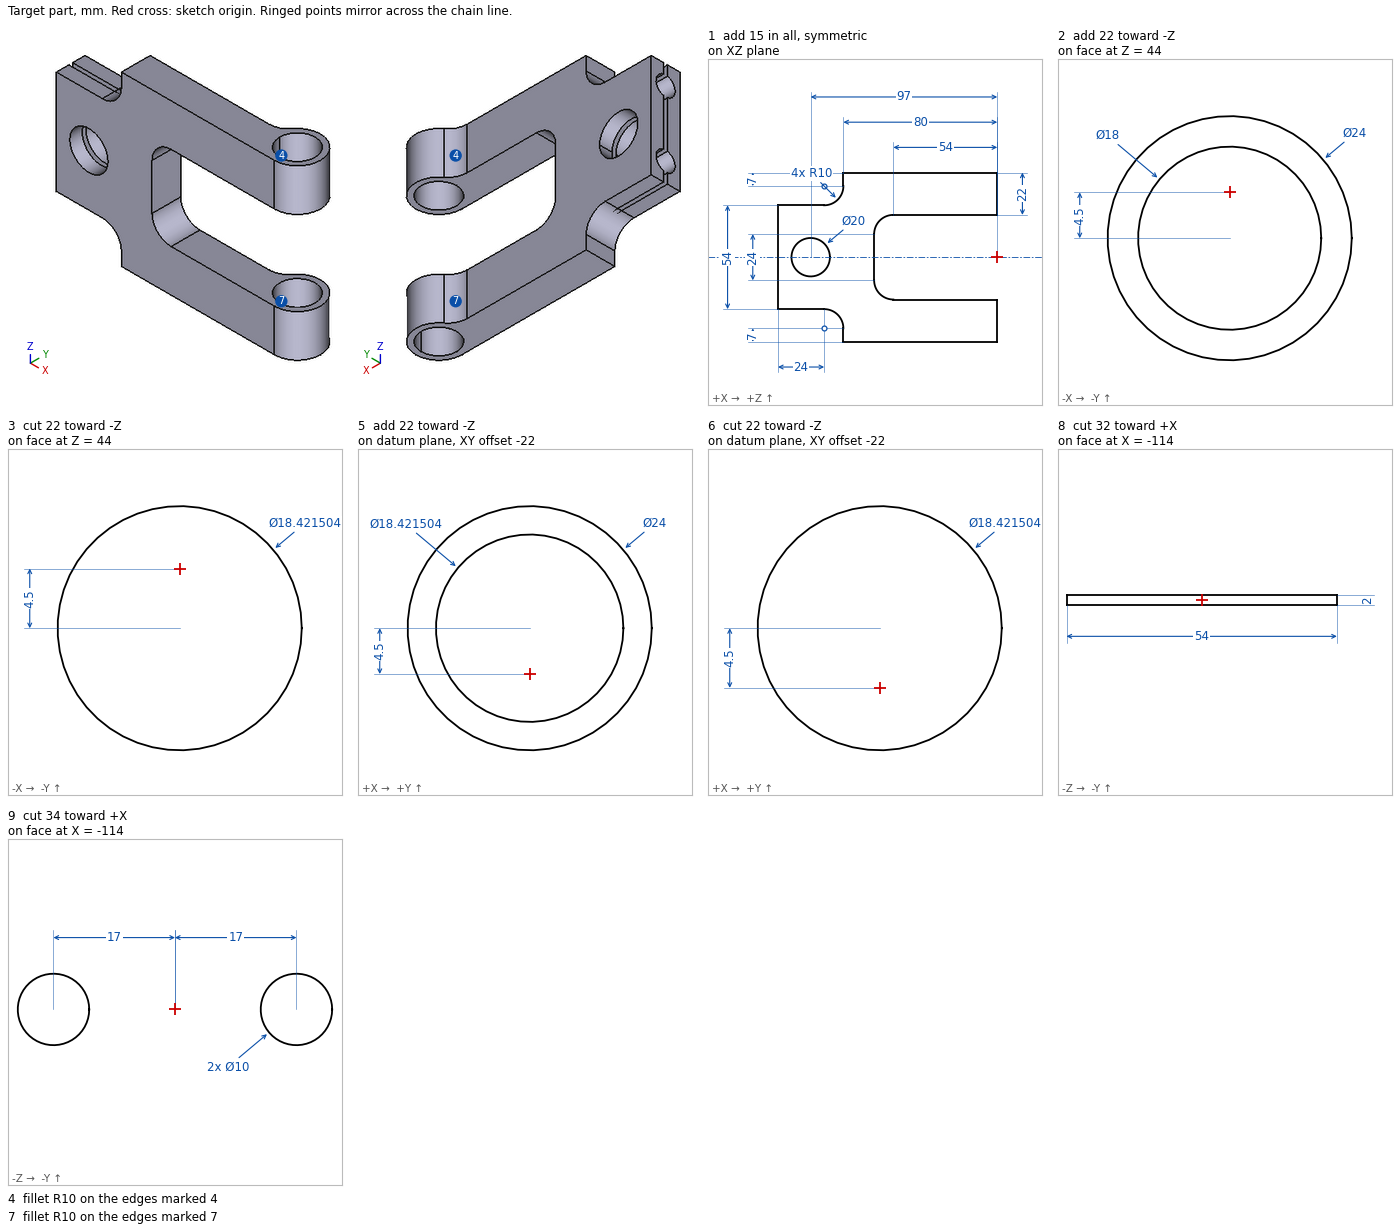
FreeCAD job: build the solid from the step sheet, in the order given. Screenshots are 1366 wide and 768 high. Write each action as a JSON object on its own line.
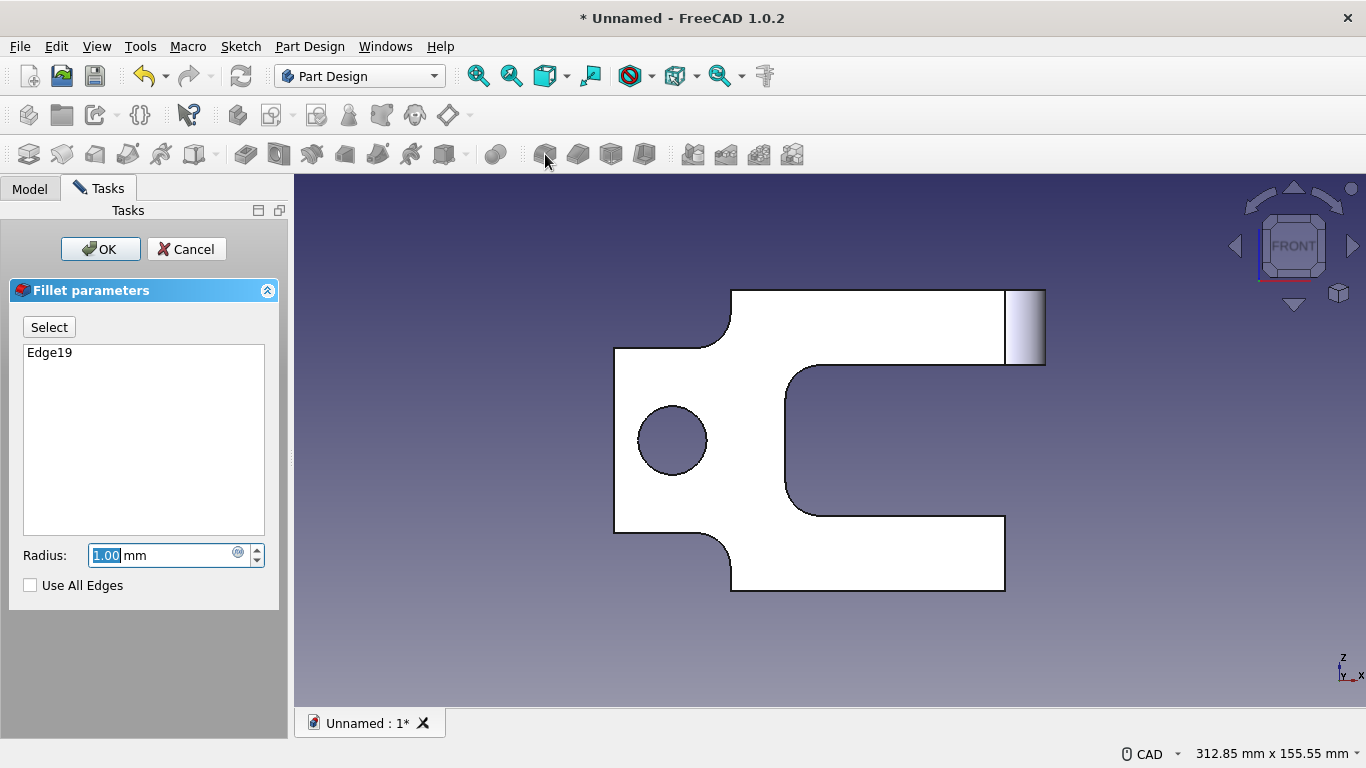
{"action": "type", "text": "10"}
{"action": "key", "text": "Tab"}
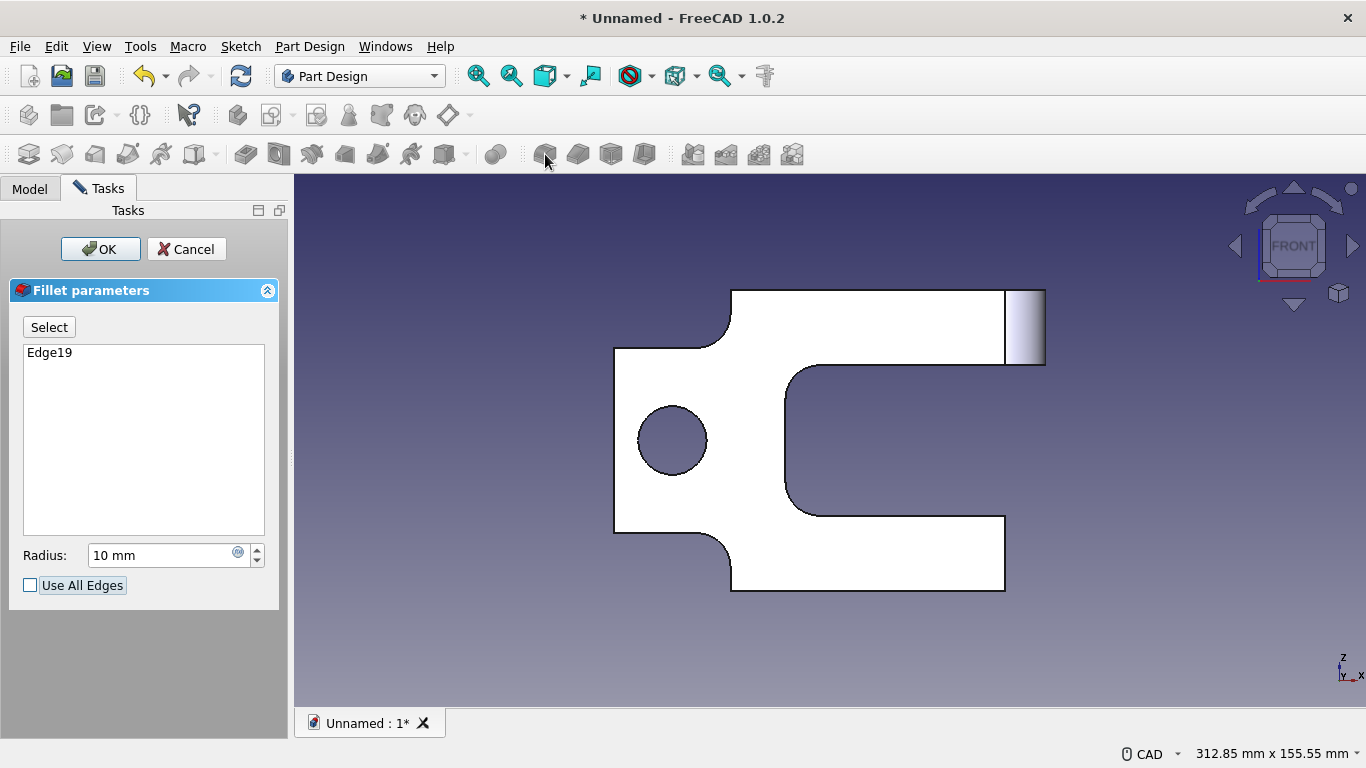
{"action": "left_click", "coordinate": [101, 249]}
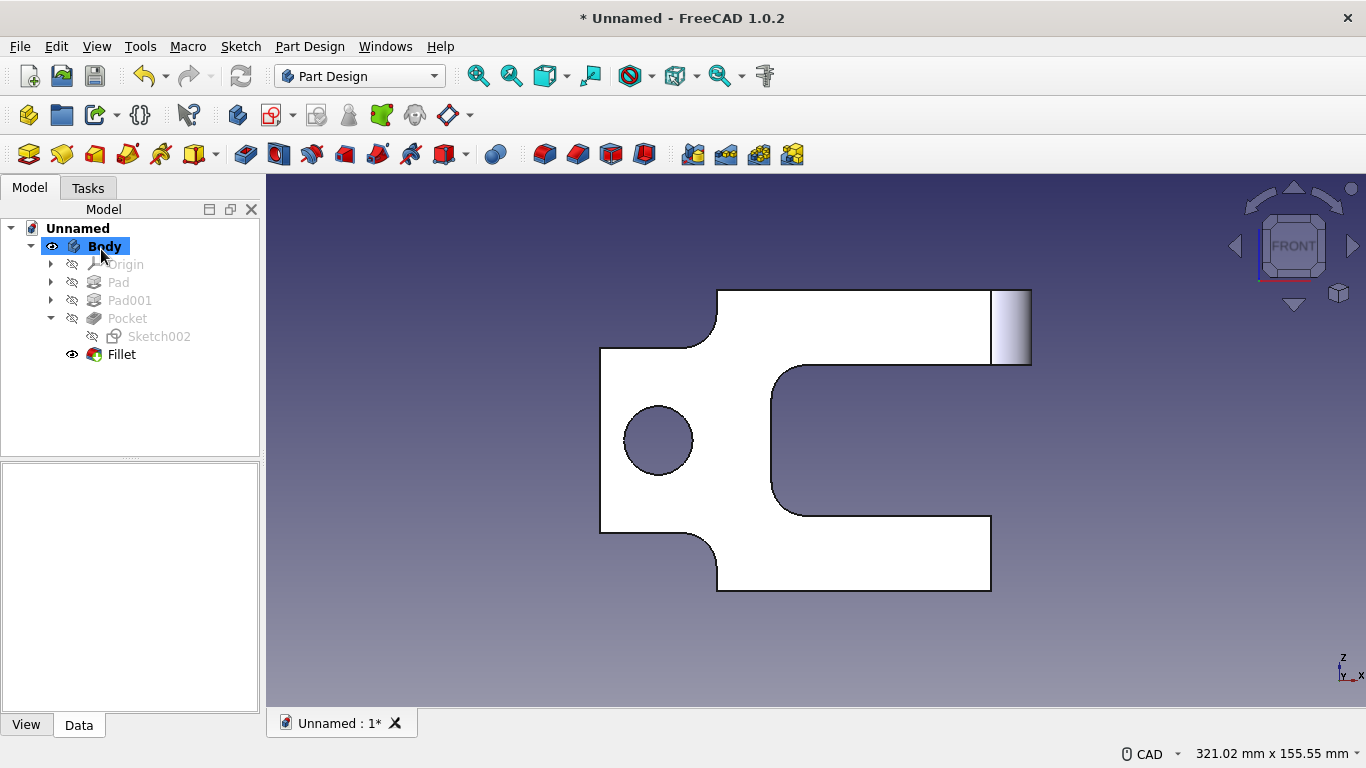
{"action": "left_click", "coordinate": [51, 264]}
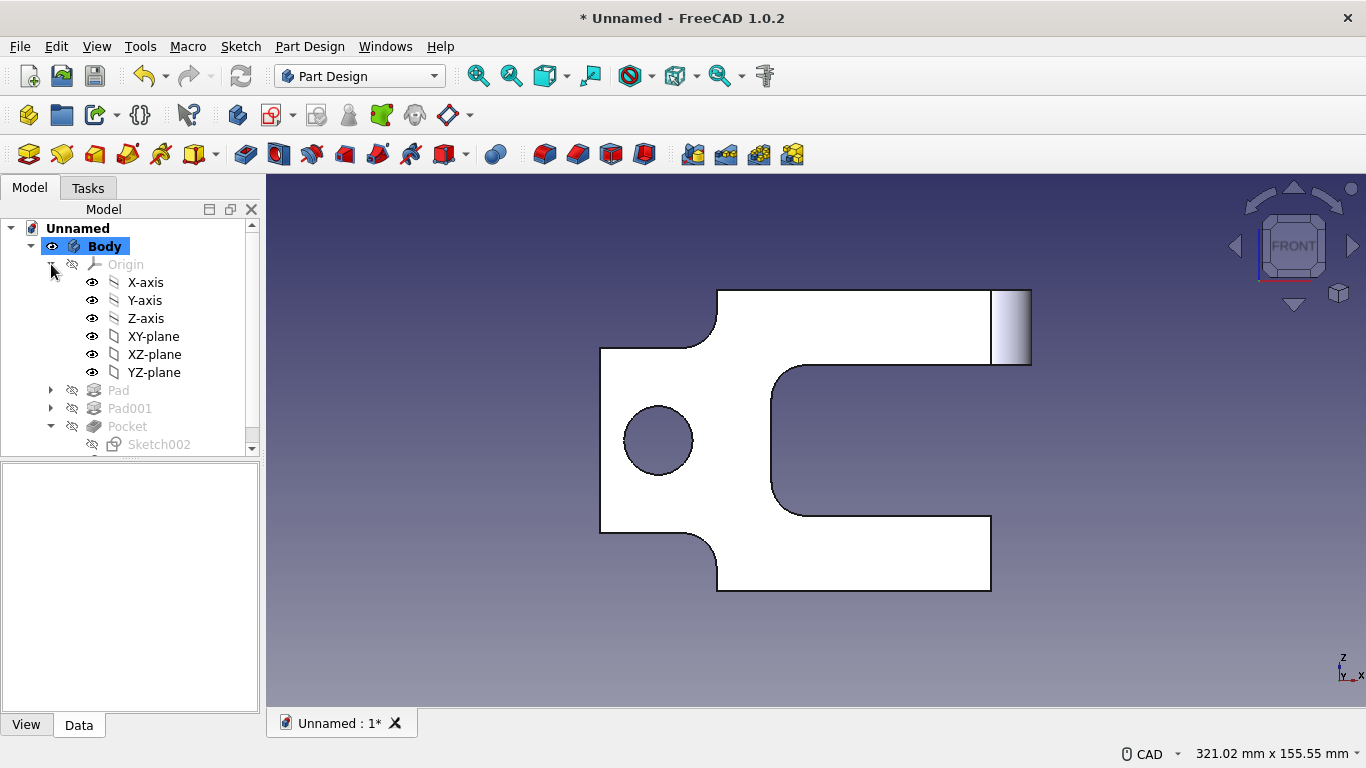
{"action": "left_click", "coordinate": [137, 336]}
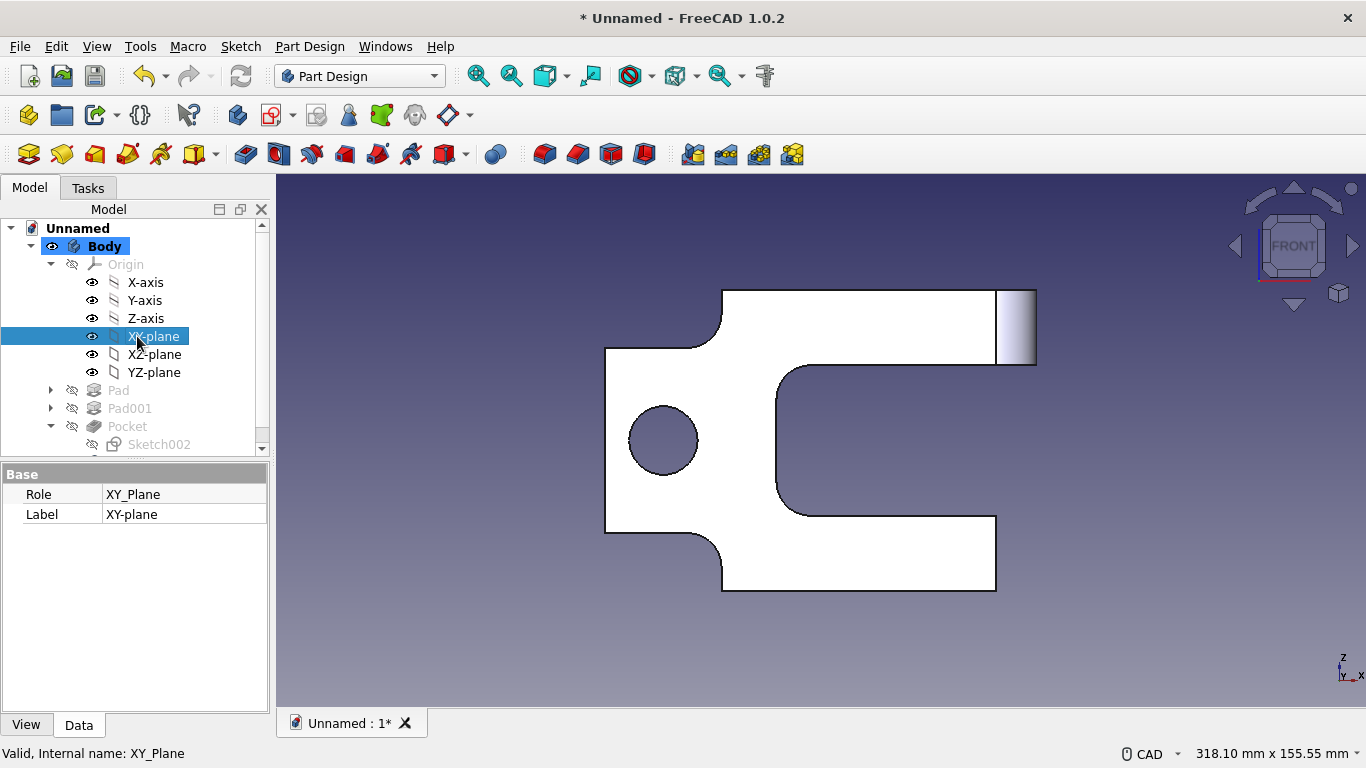
{"action": "left_click", "coordinate": [448, 116]}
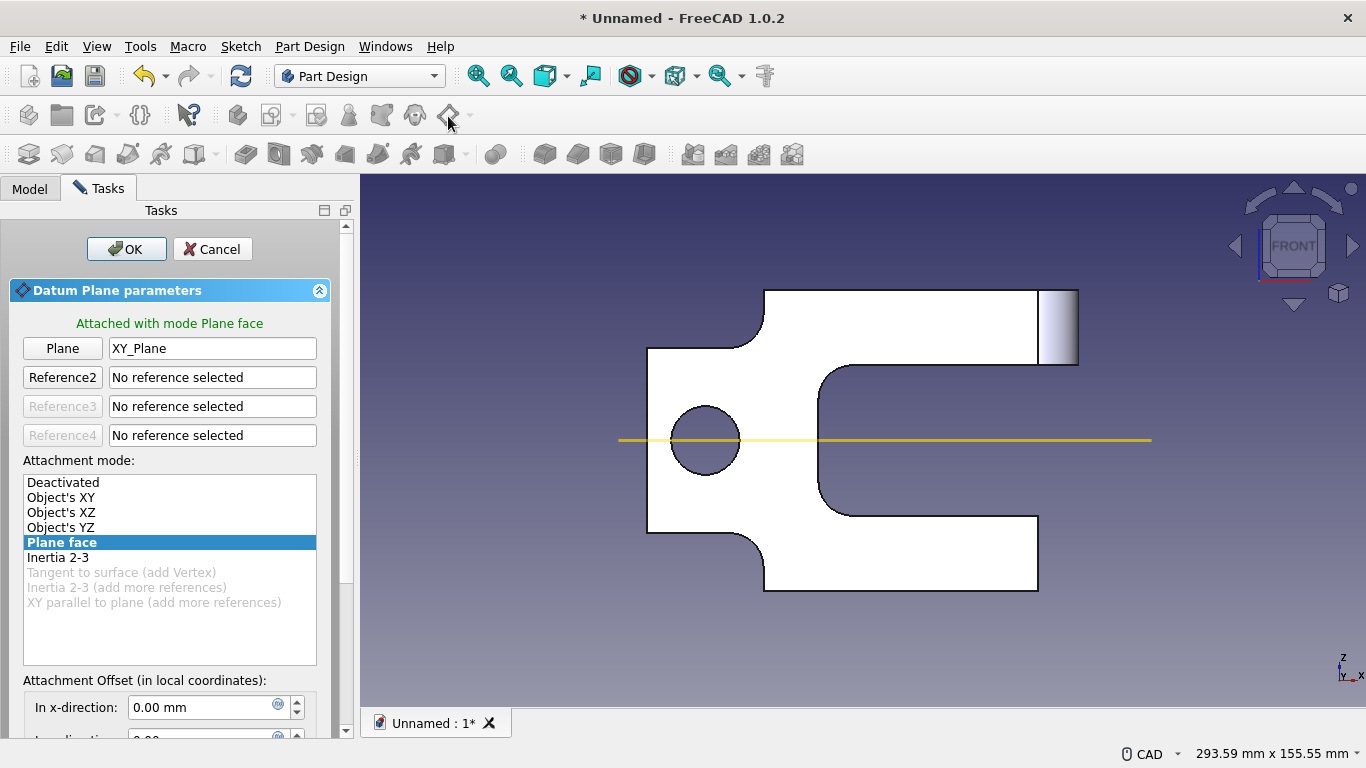
{"action": "scroll", "coordinate": [346, 479], "scroll_direction": "down", "scroll_amount": 2}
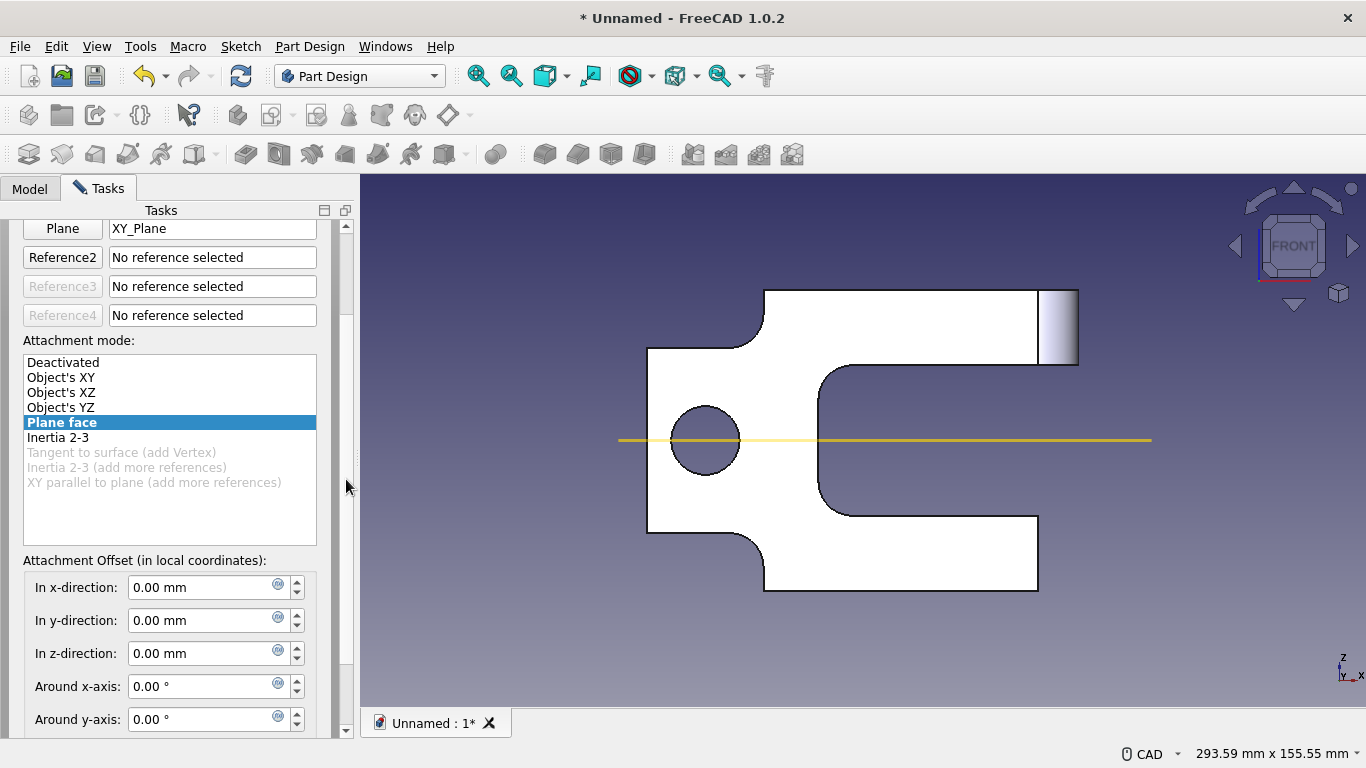
{"action": "triple_click", "coordinate": [210, 654]}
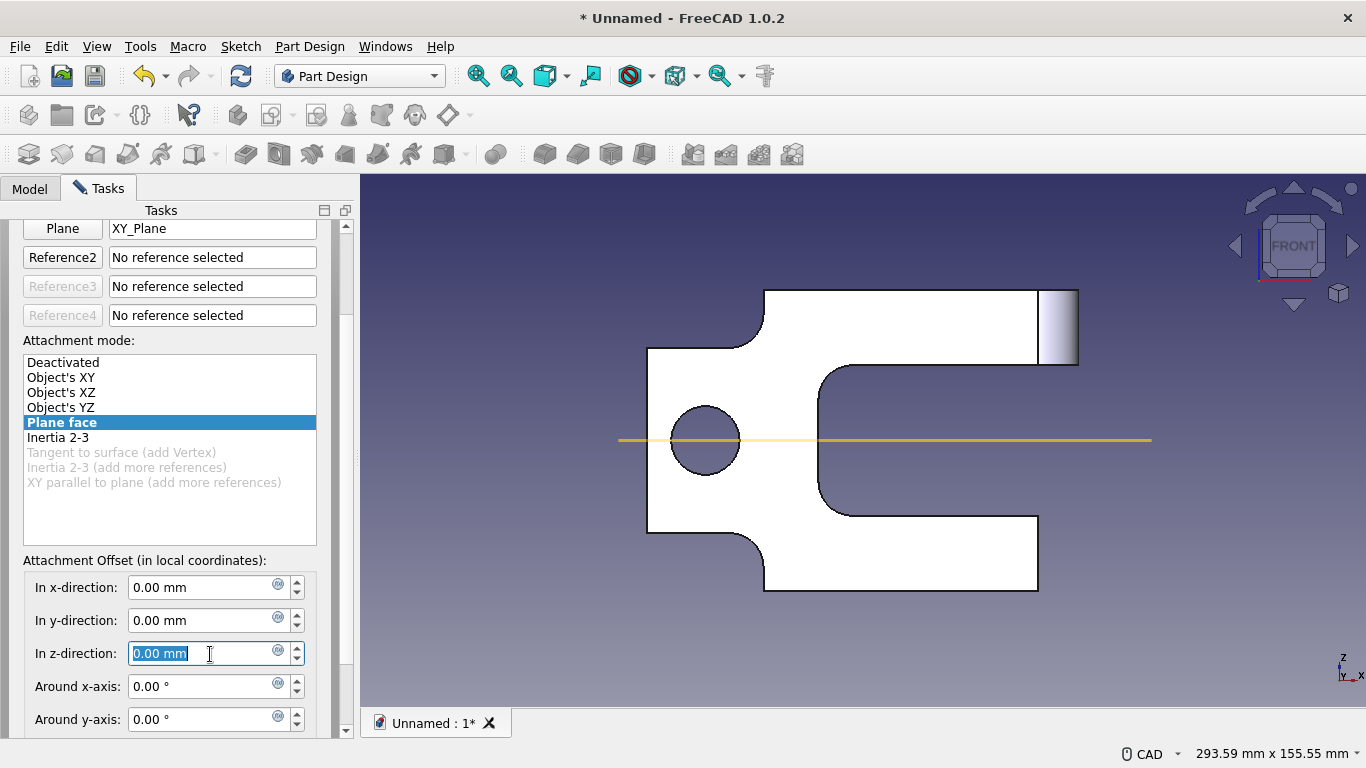
{"action": "type", "text": "-22"}
{"action": "key", "text": "Tab"}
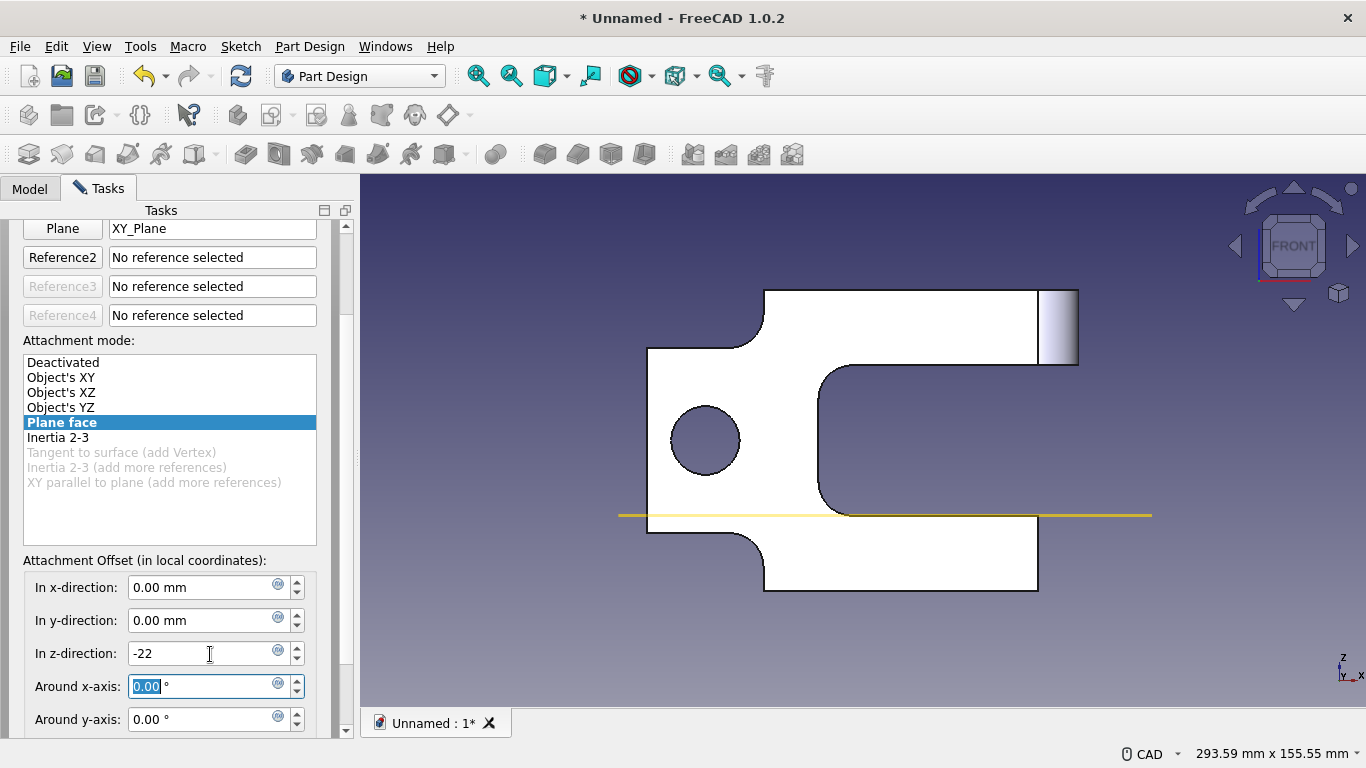
{"action": "scroll", "coordinate": [346, 479], "scroll_direction": "up", "scroll_amount": 3}